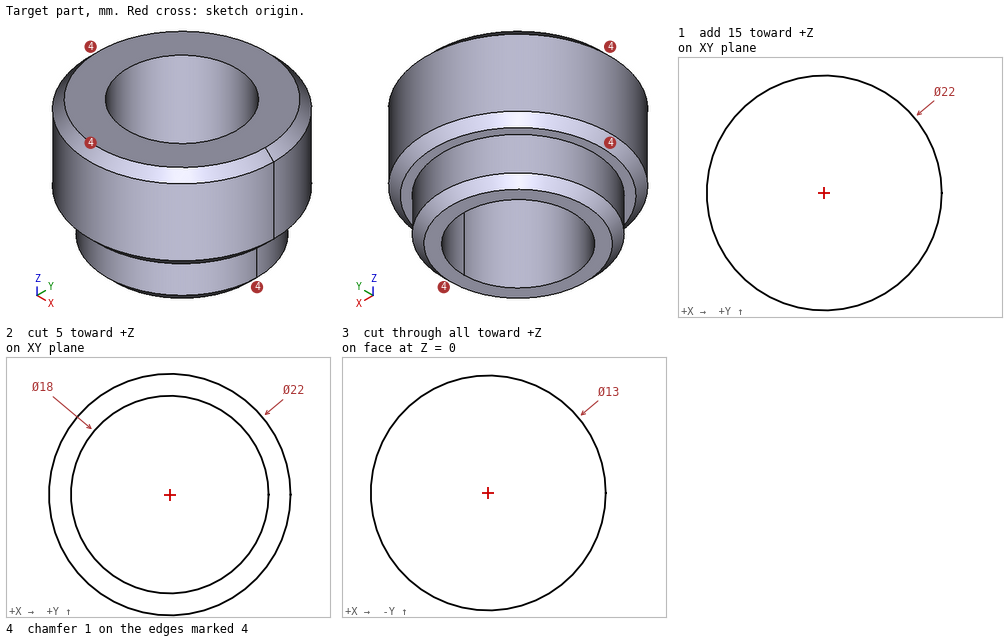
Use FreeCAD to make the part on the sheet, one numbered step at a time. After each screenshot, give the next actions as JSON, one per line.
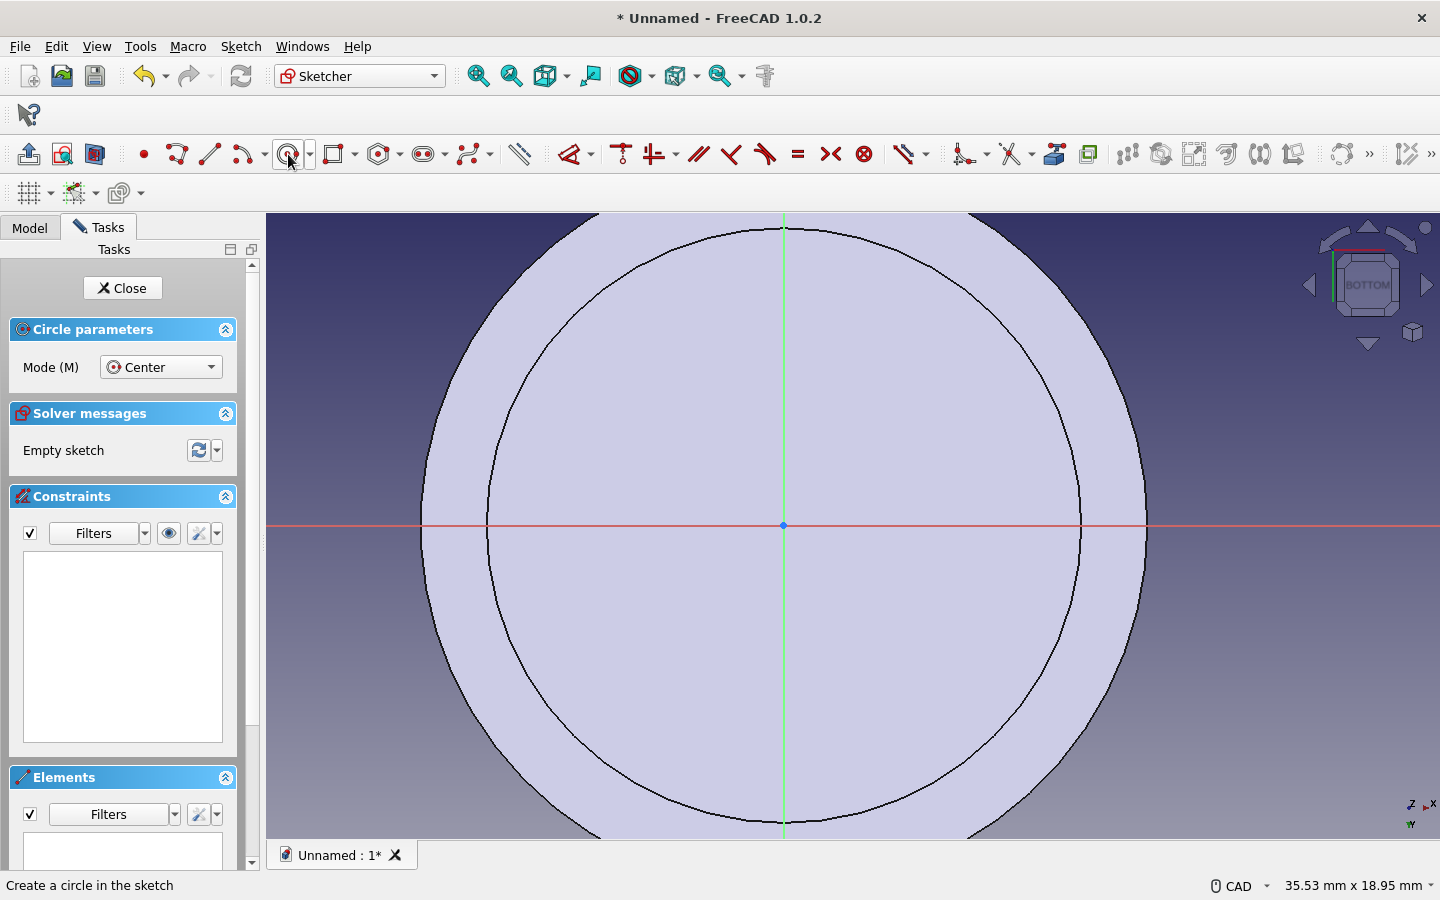
{"action": "left_click", "coordinate": [784, 526]}
{"action": "mouse_move", "coordinate": [936, 374]}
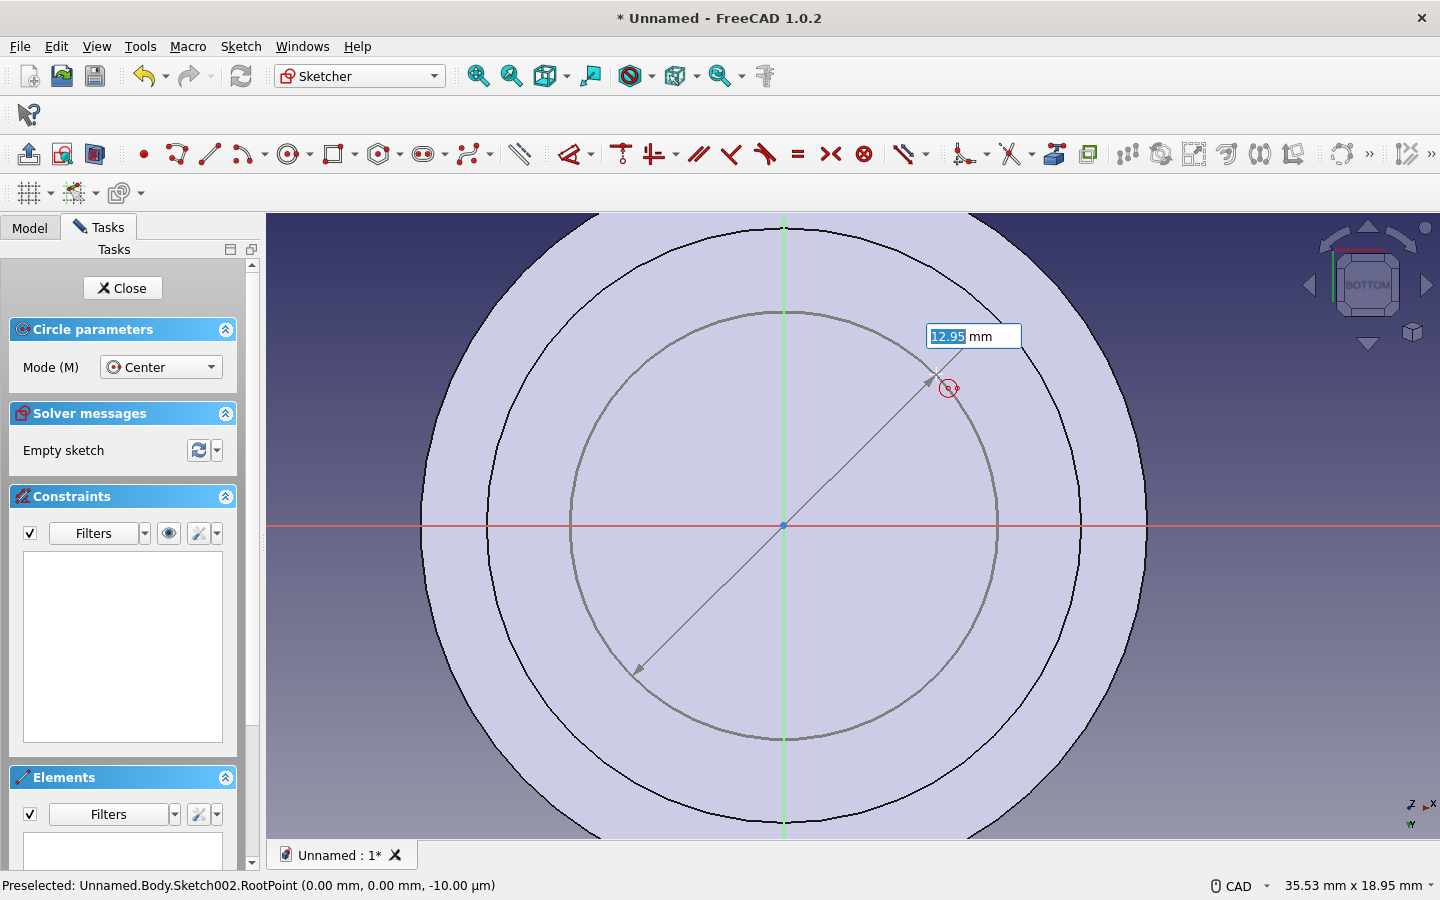
{"action": "type", "text": "13"}
{"action": "key", "text": "Return"}
{"action": "key", "text": "Escape"}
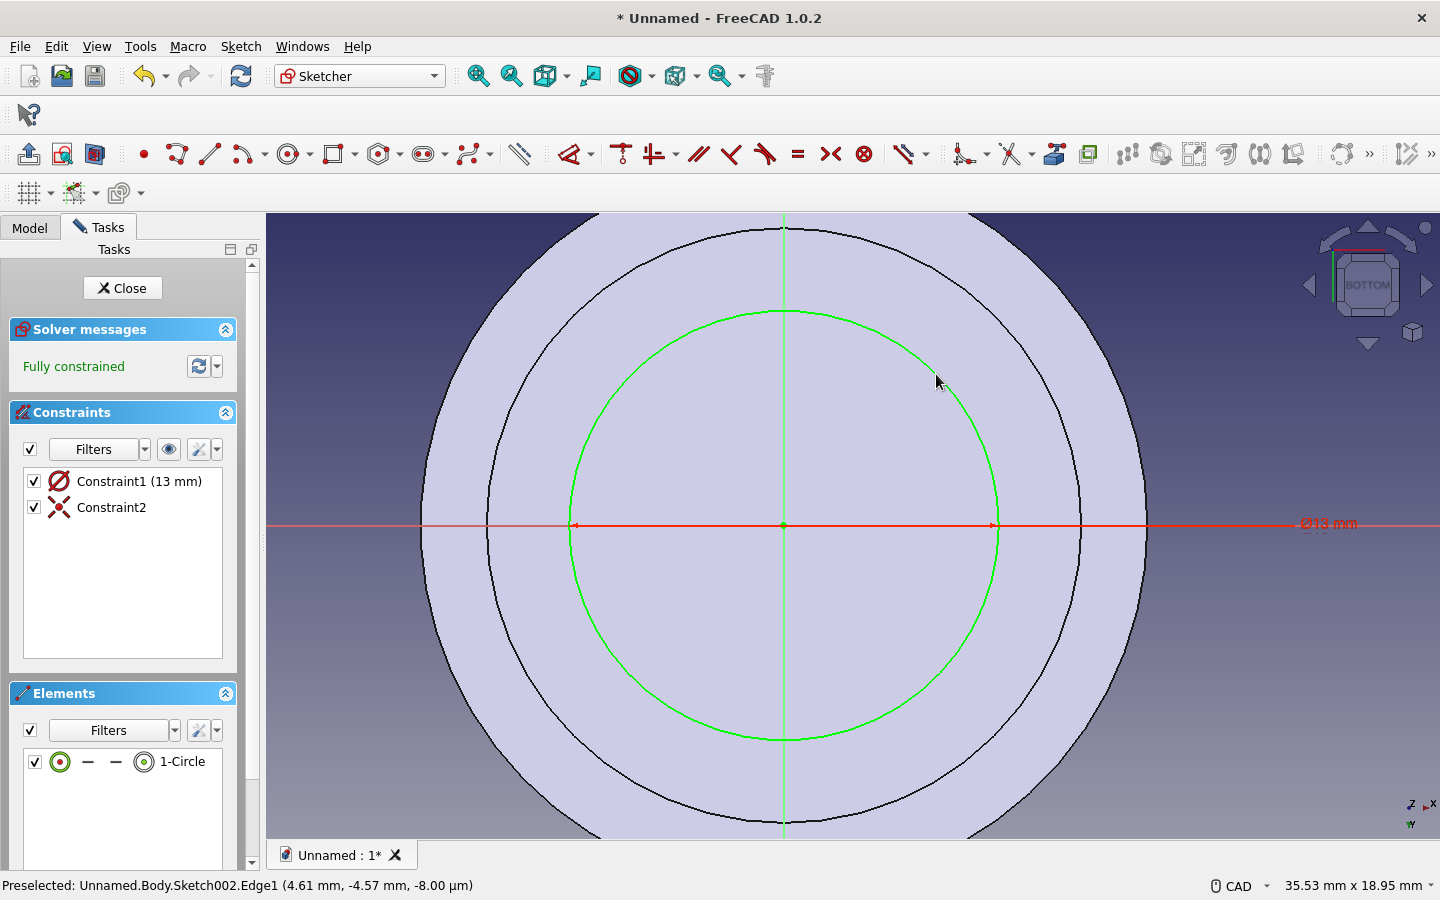
{"action": "left_click", "coordinate": [123, 288]}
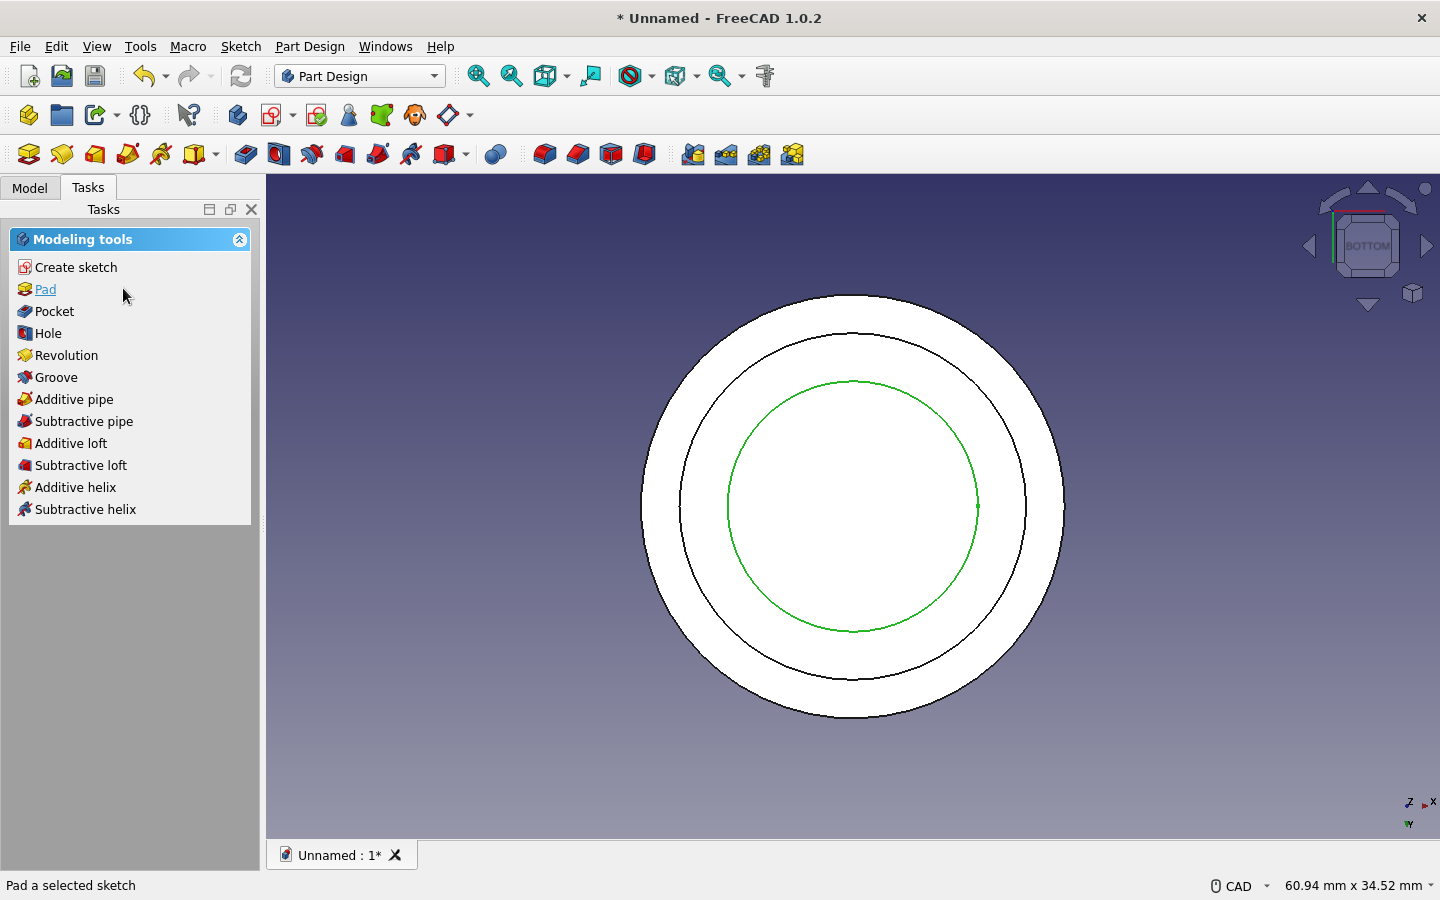
{"action": "left_click", "coordinate": [246, 154]}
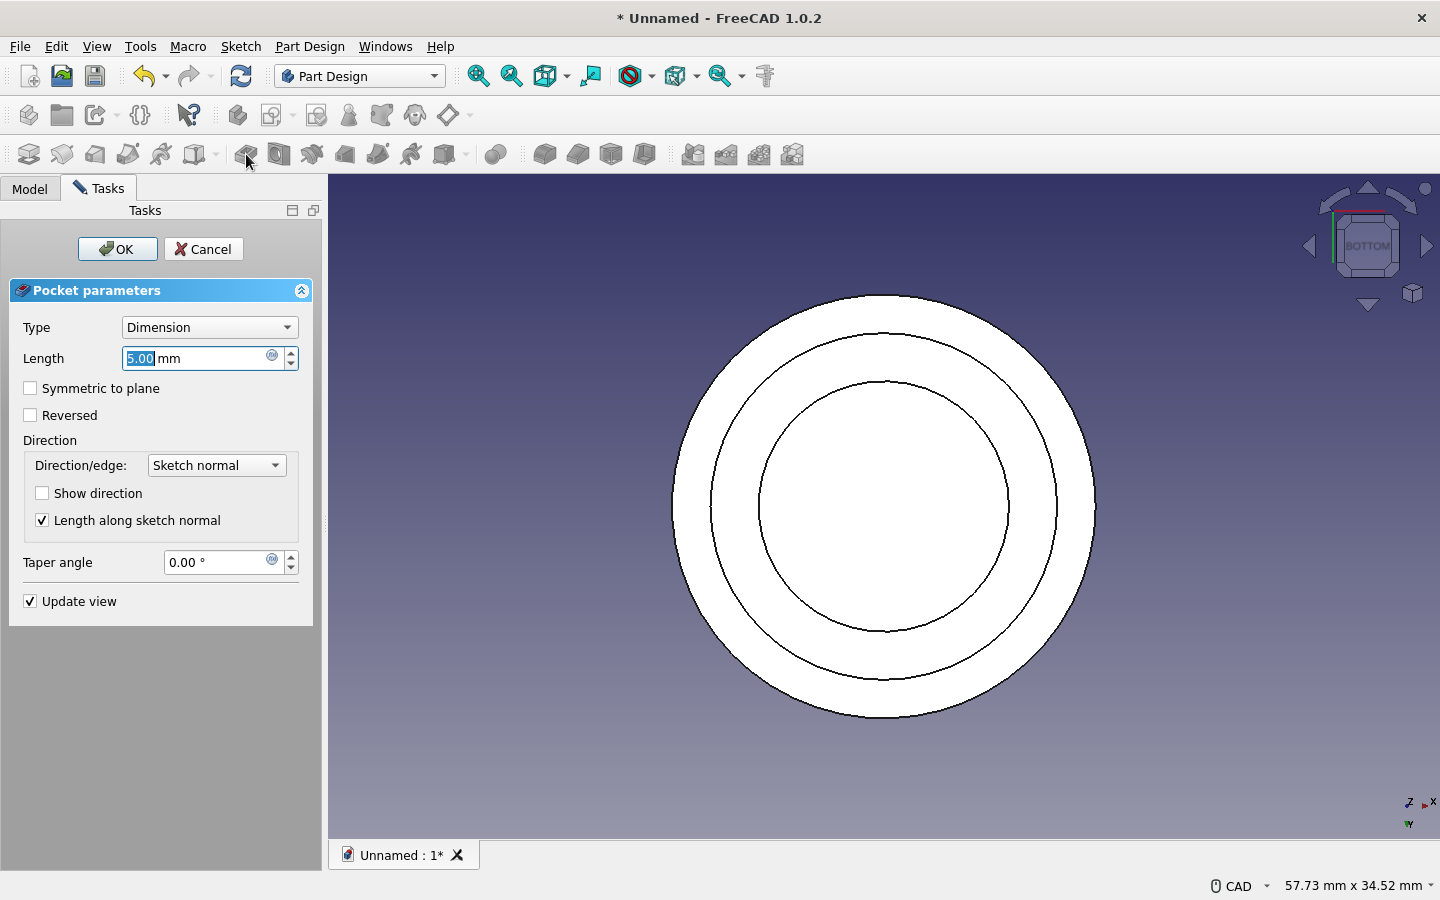
{"action": "left_click", "coordinate": [210, 328]}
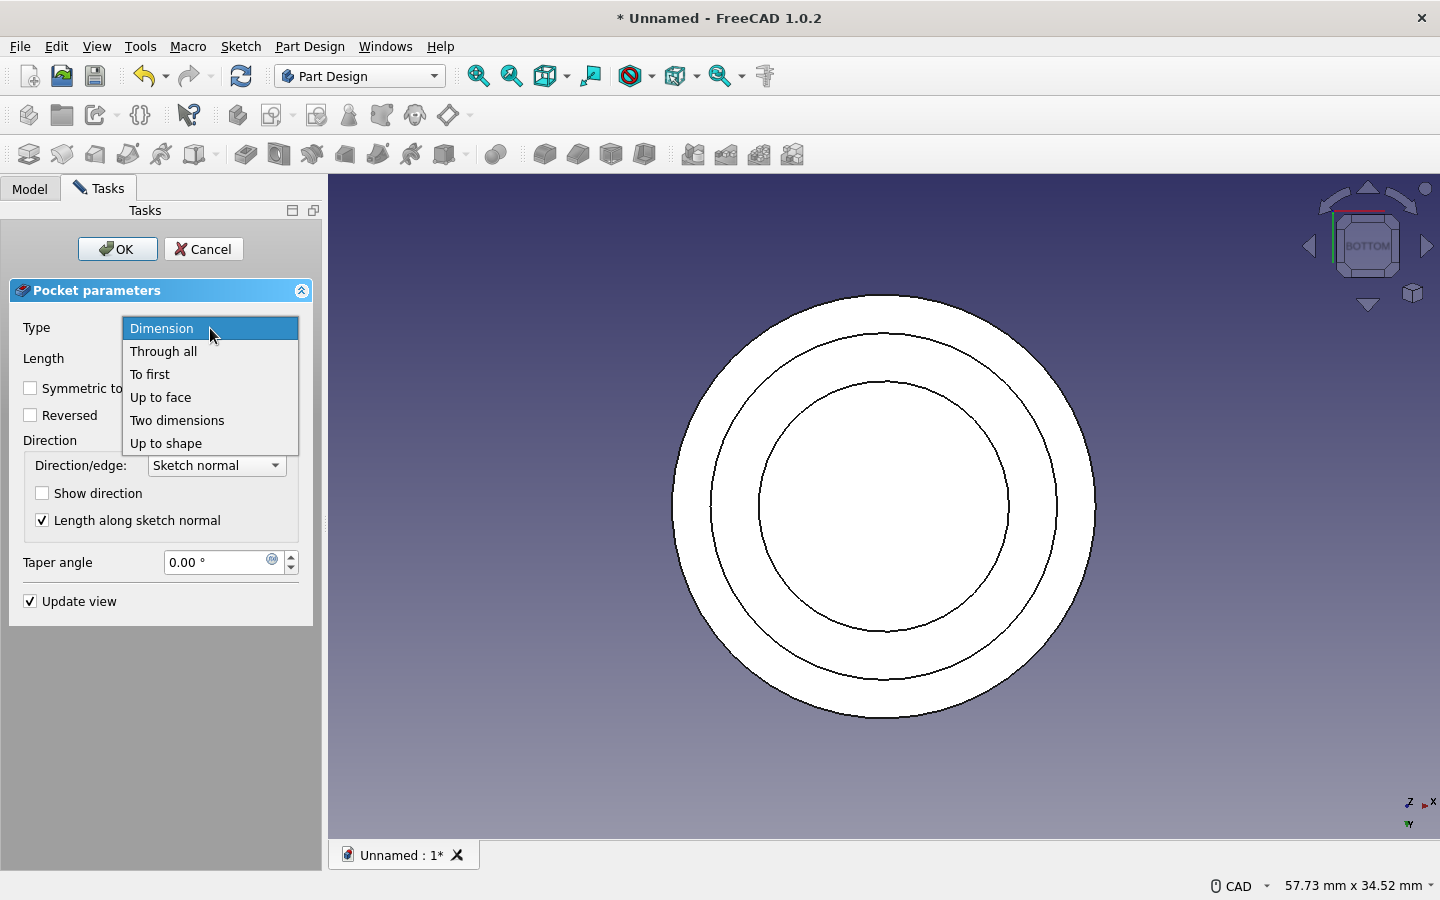
{"action": "left_click", "coordinate": [208, 352]}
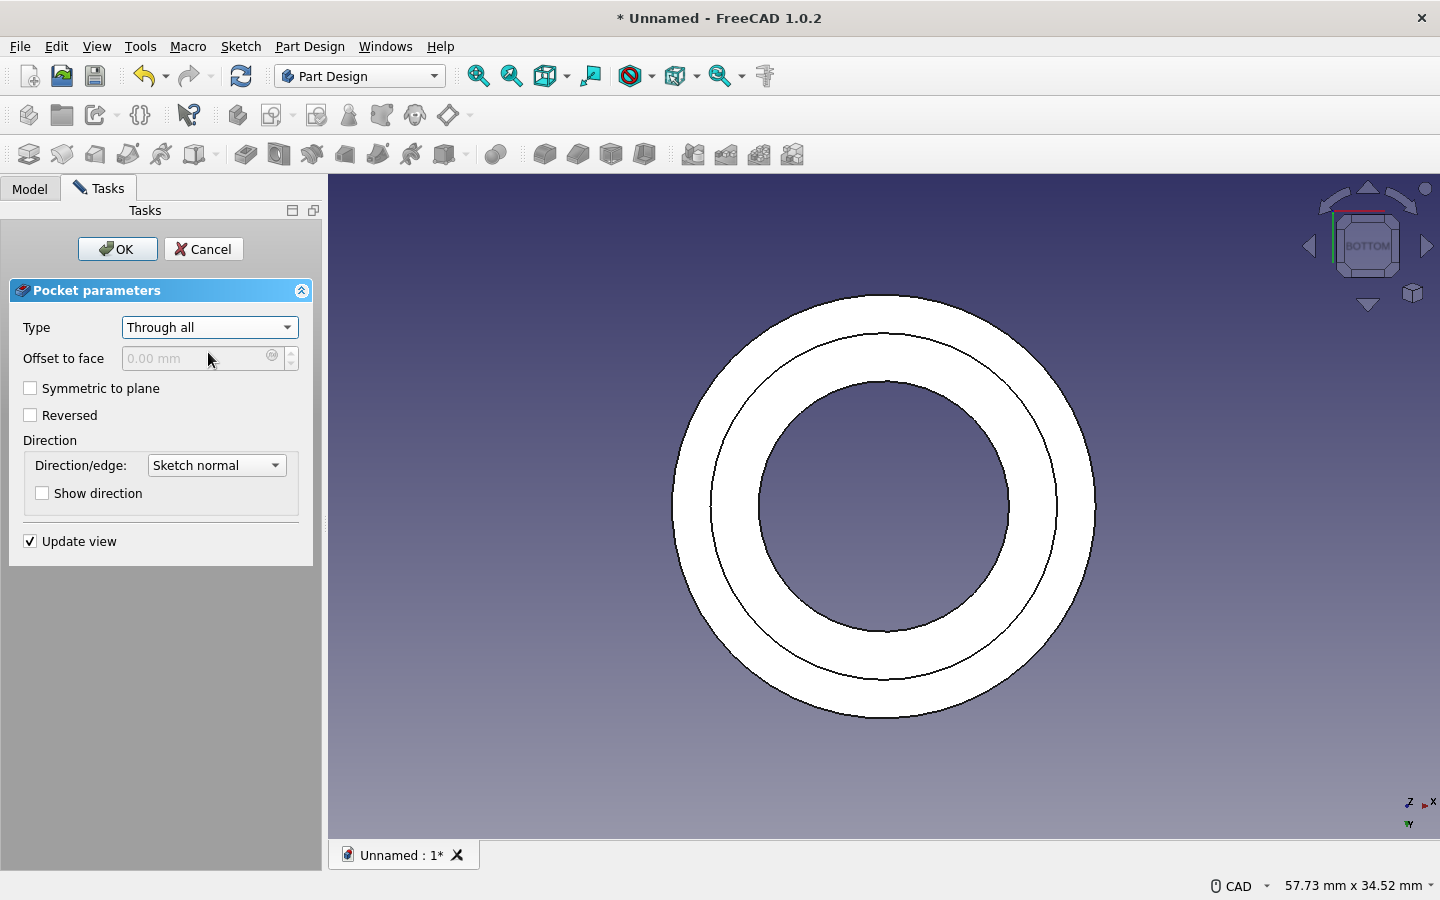
{"action": "left_click", "coordinate": [118, 249]}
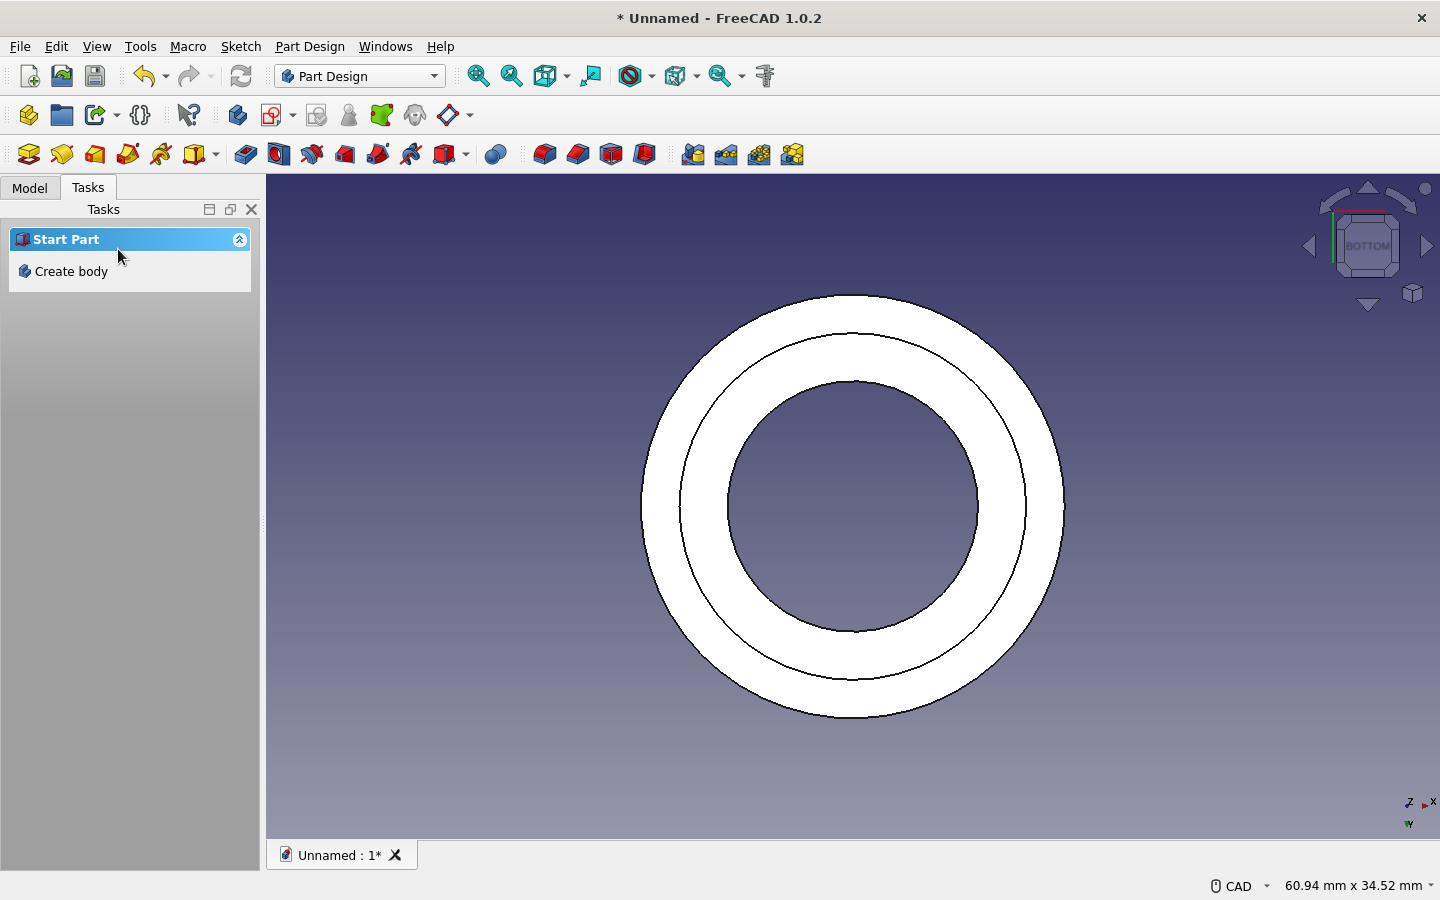
{"action": "left_click", "coordinate": [641, 506]}